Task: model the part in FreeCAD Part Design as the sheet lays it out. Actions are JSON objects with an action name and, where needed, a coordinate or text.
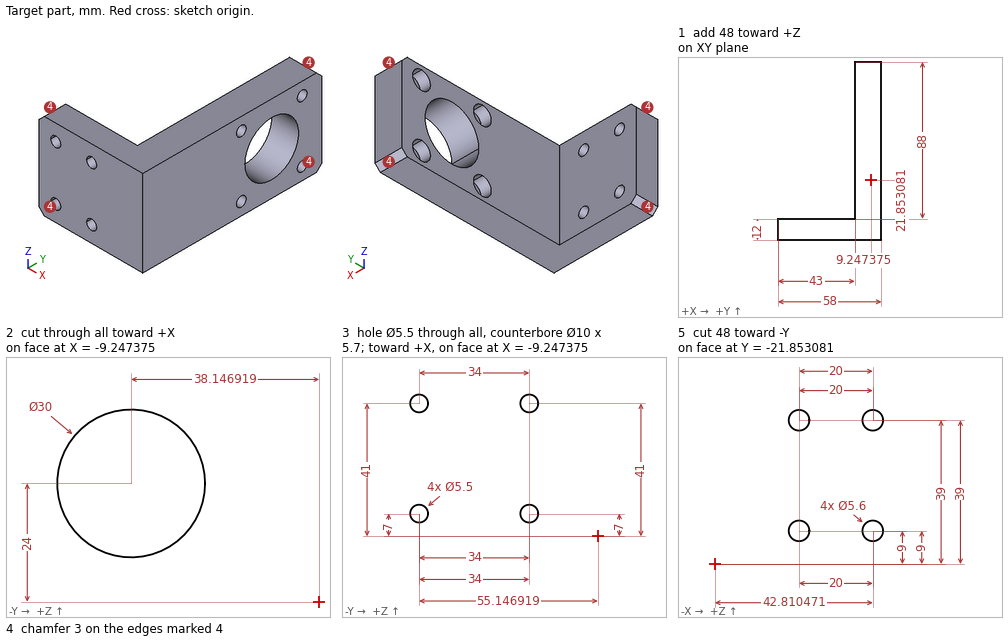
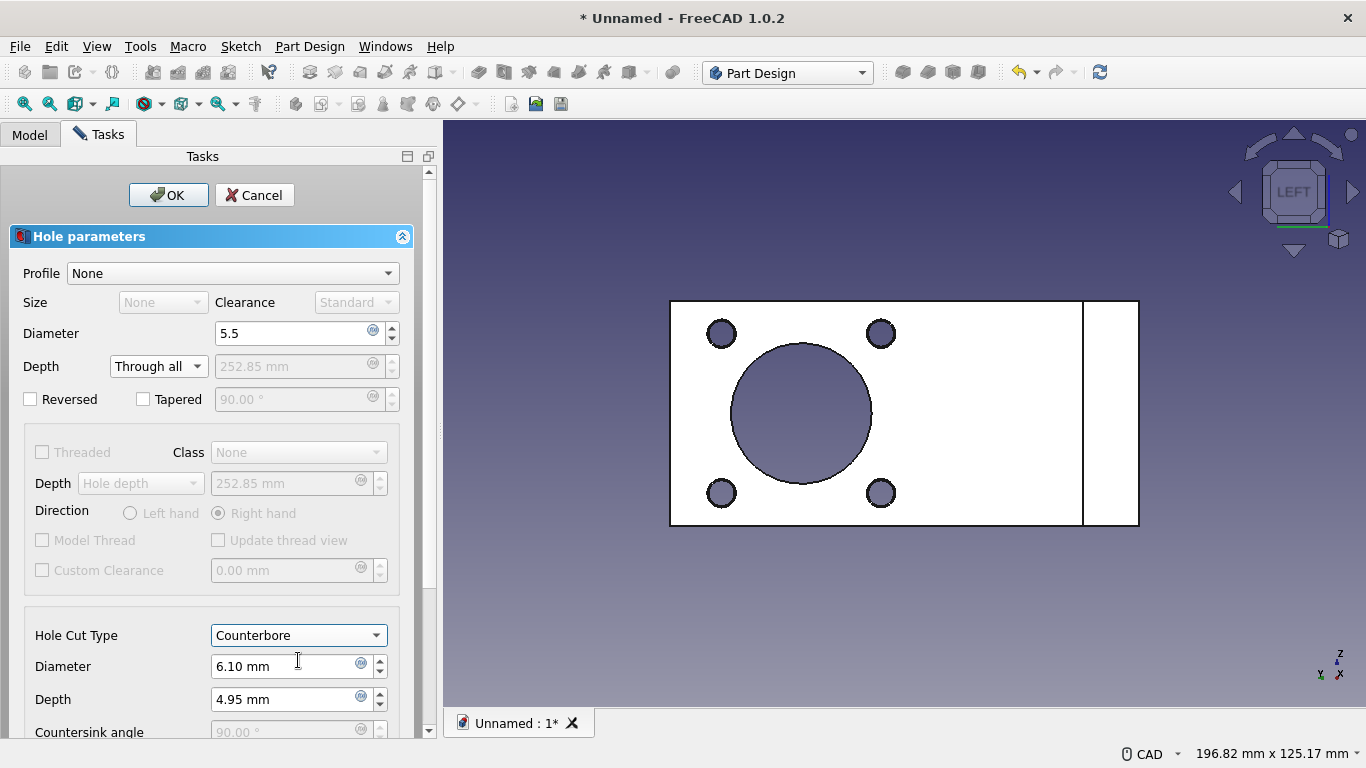
{"action": "triple_click", "coordinate": [292, 666]}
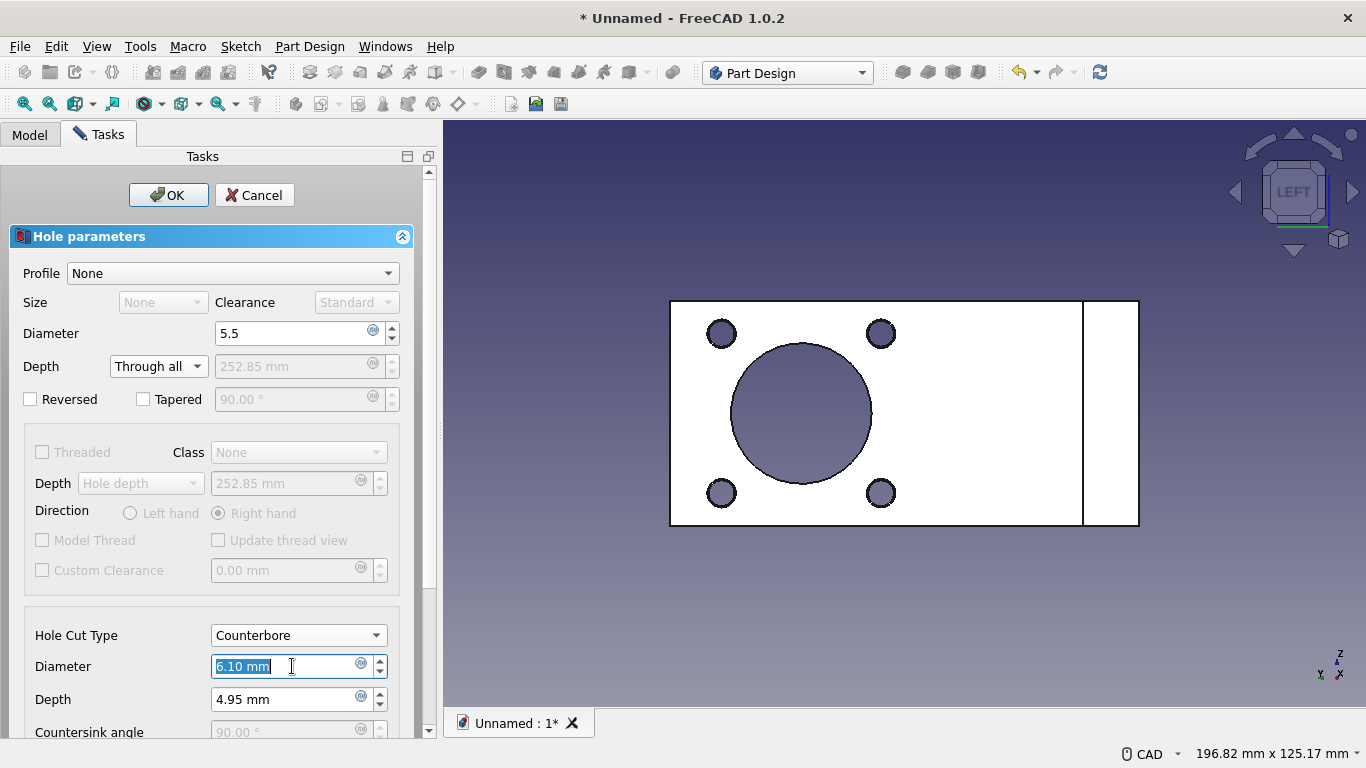
{"action": "type", "text": "10"}
{"action": "key", "text": "Tab"}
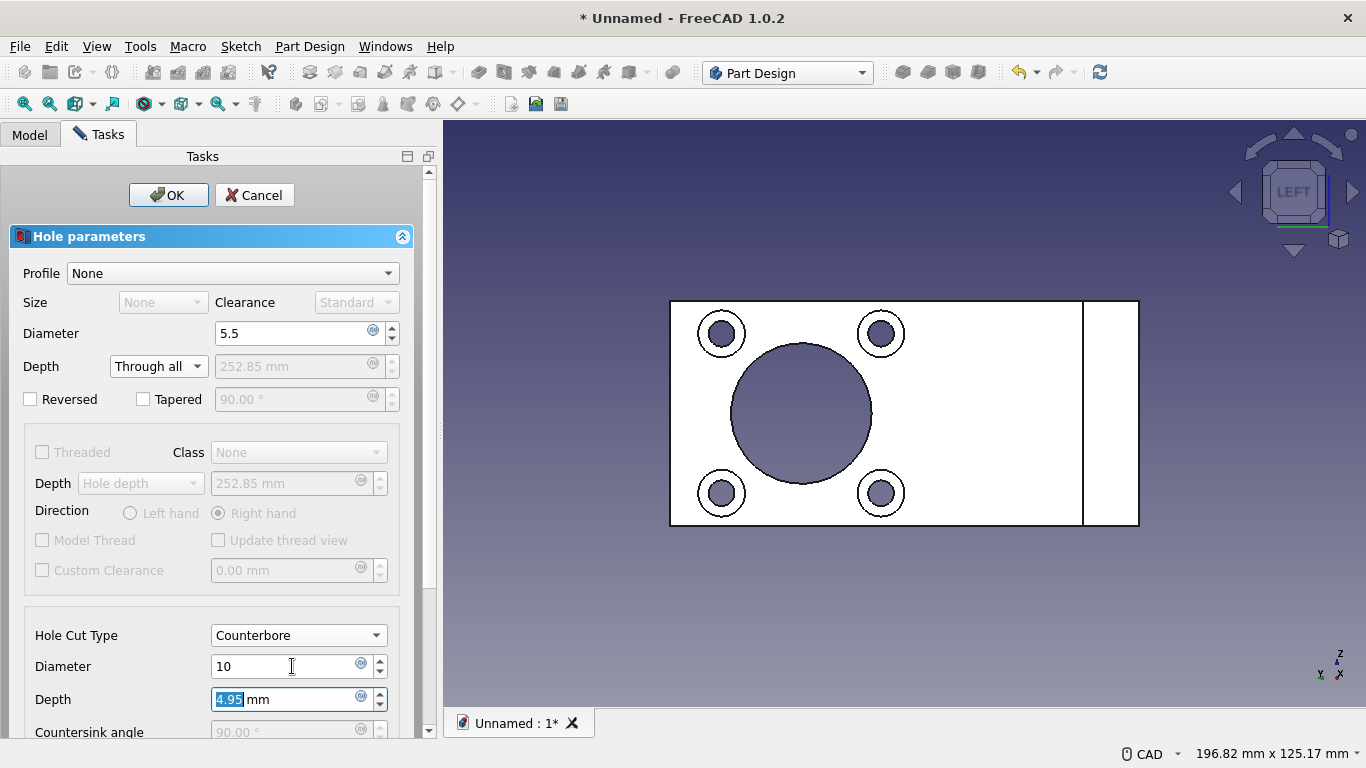
{"action": "type", "text": "5.7"}
{"action": "key", "text": "Tab"}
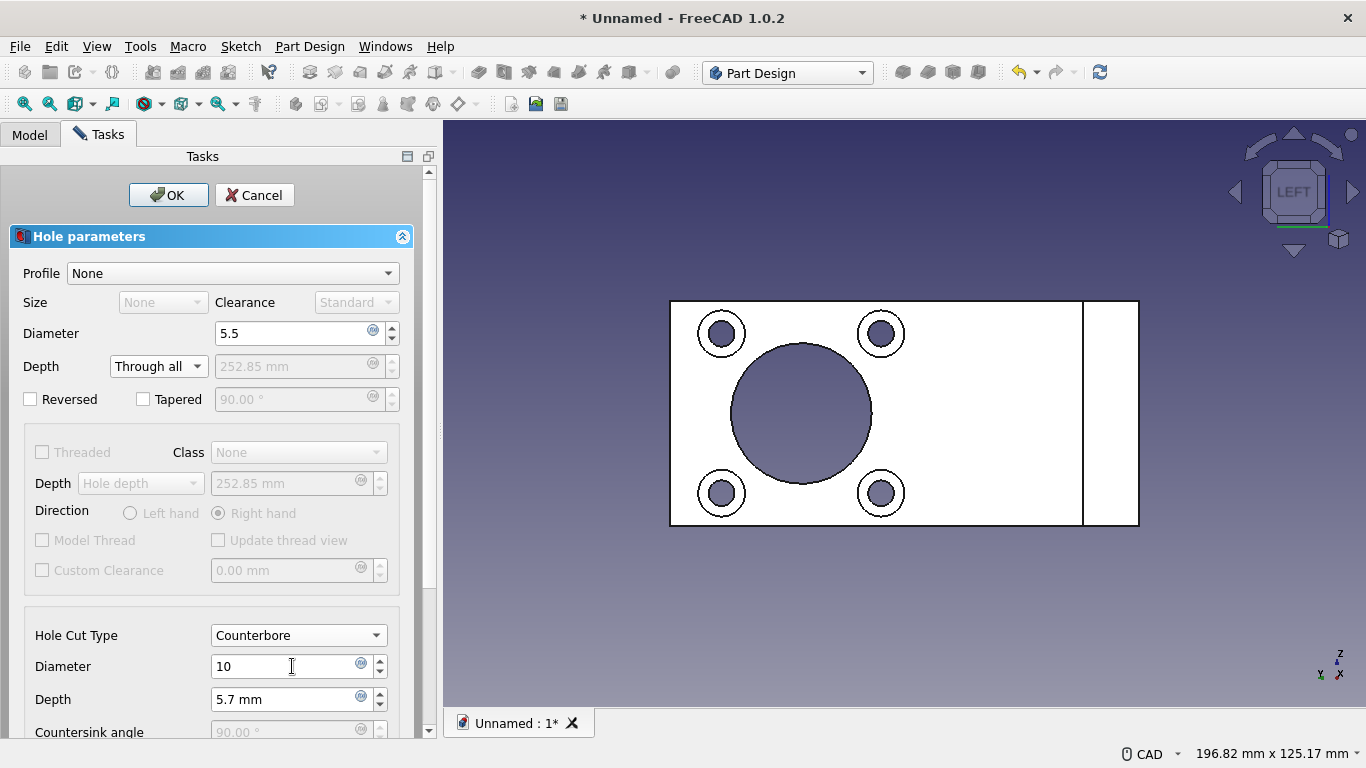
{"action": "left_click", "coordinate": [169, 195]}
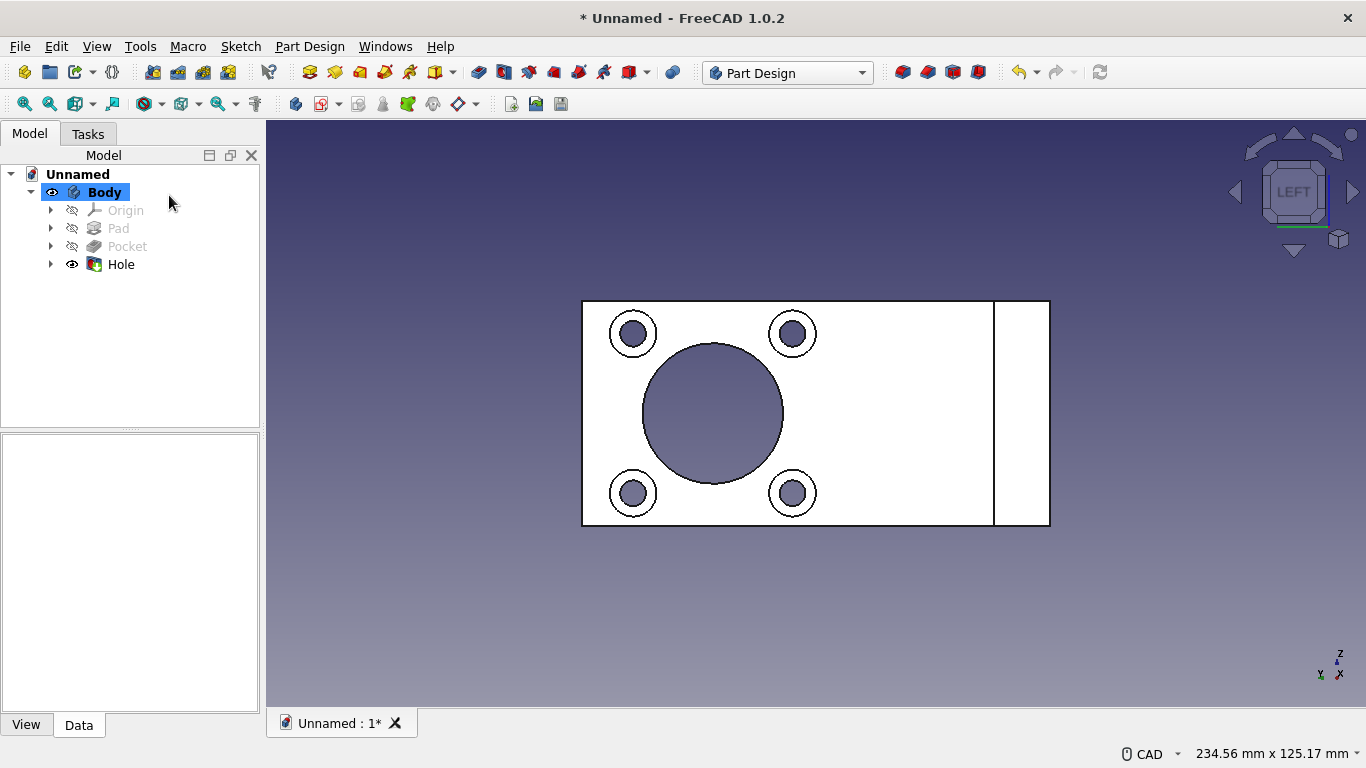
{"action": "left_click", "coordinate": [25, 104]}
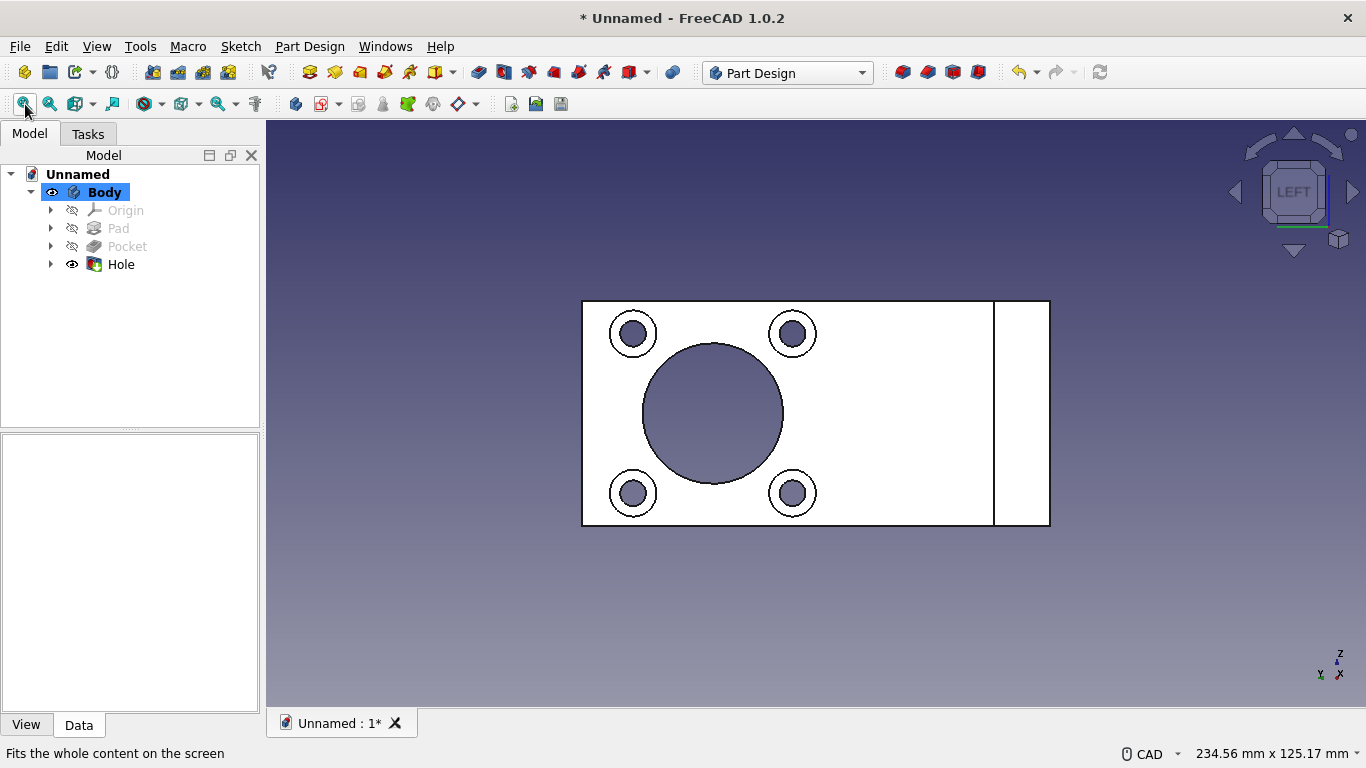
{"action": "left_click", "coordinate": [1022, 300]}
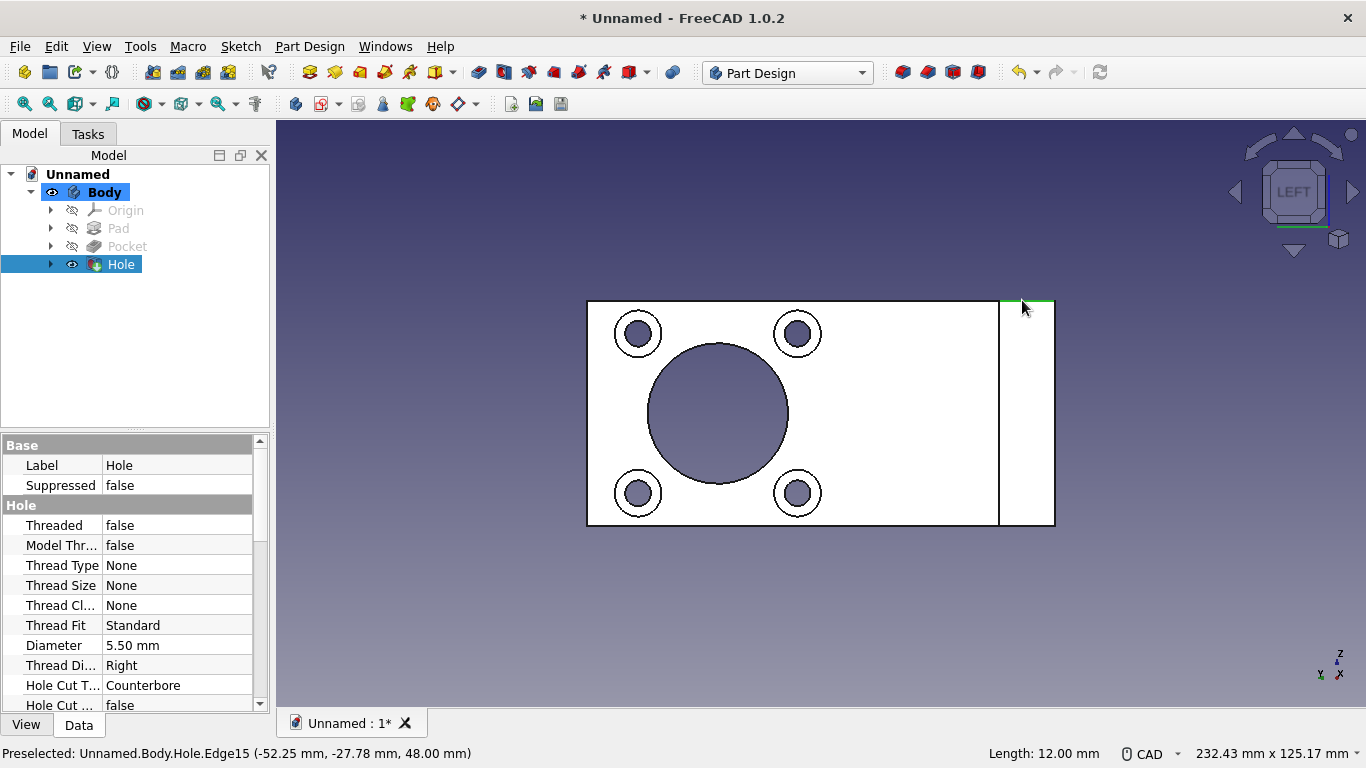
{"action": "left_click", "coordinate": [1027, 525], "text": "ctrl"}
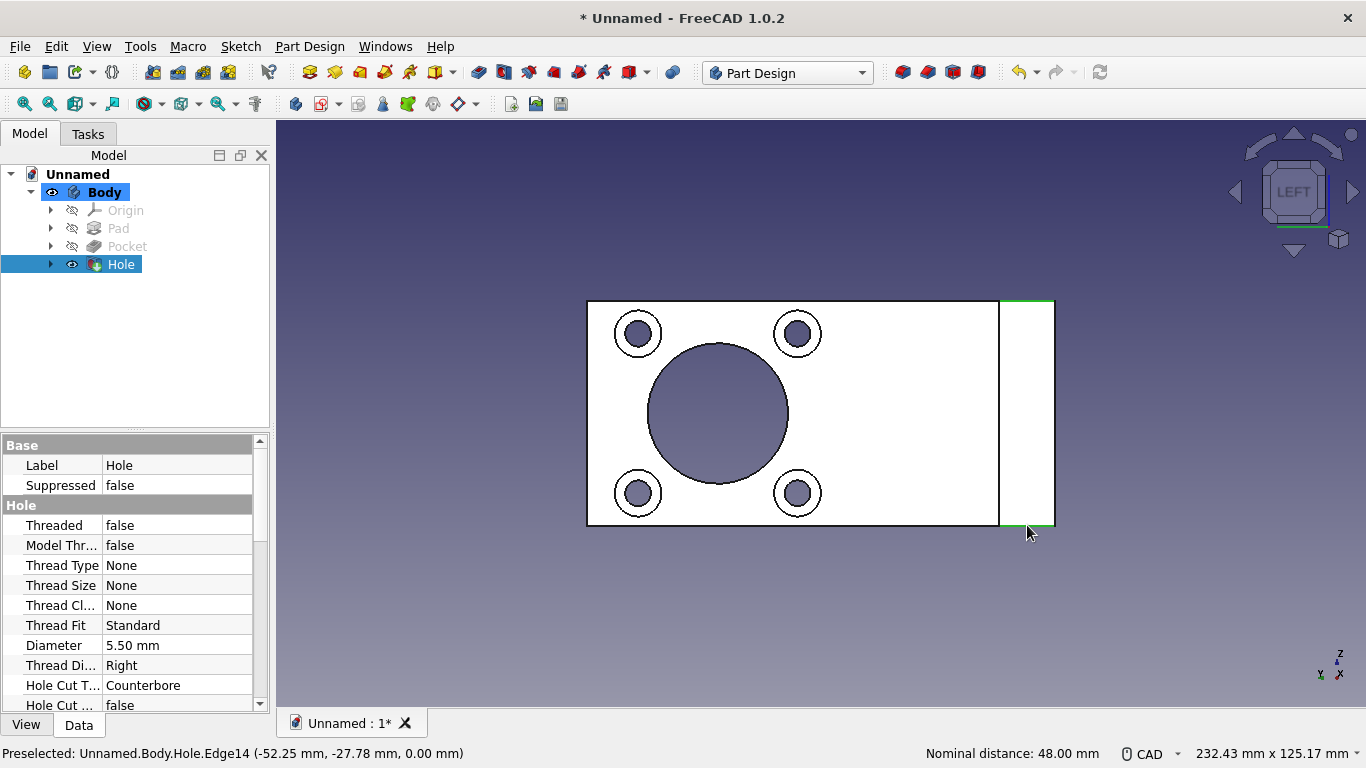
{"action": "key", "text": "0"}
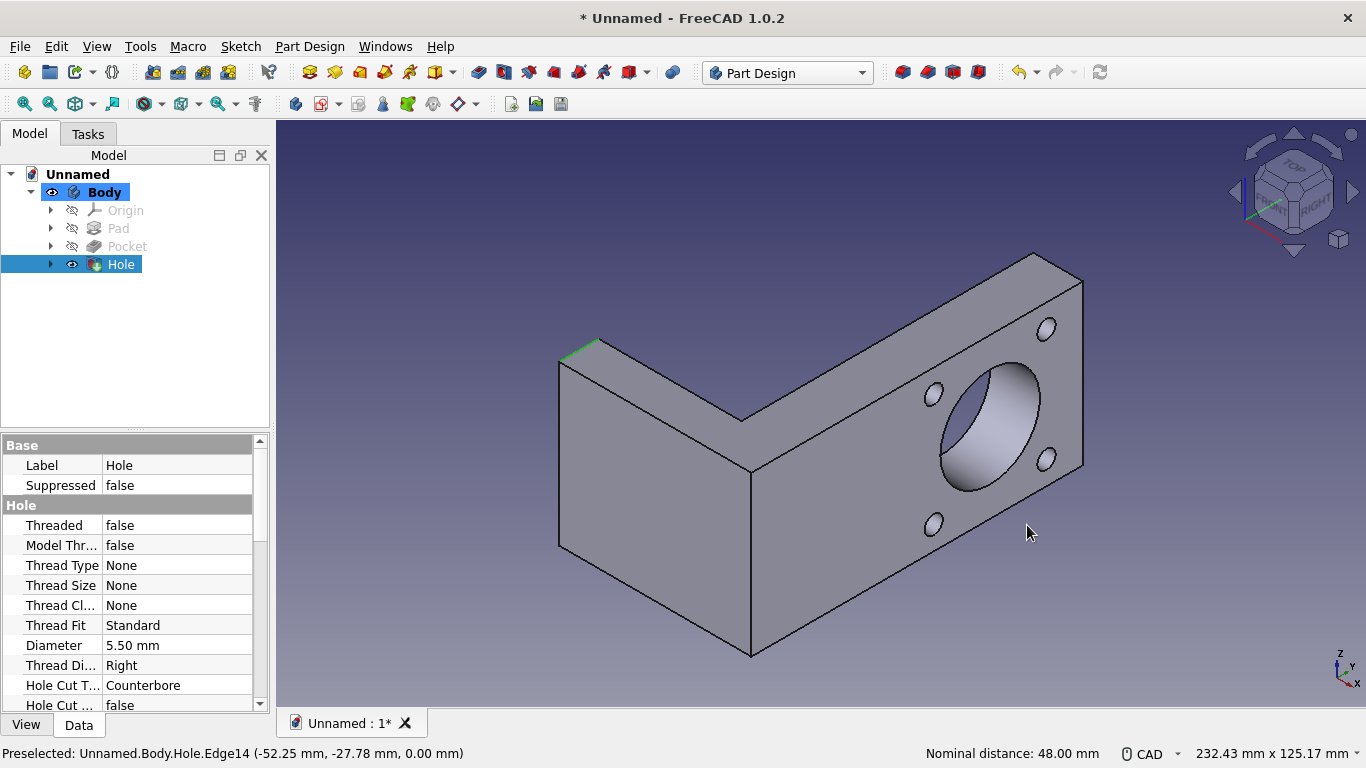
{"action": "key", "text": "2"}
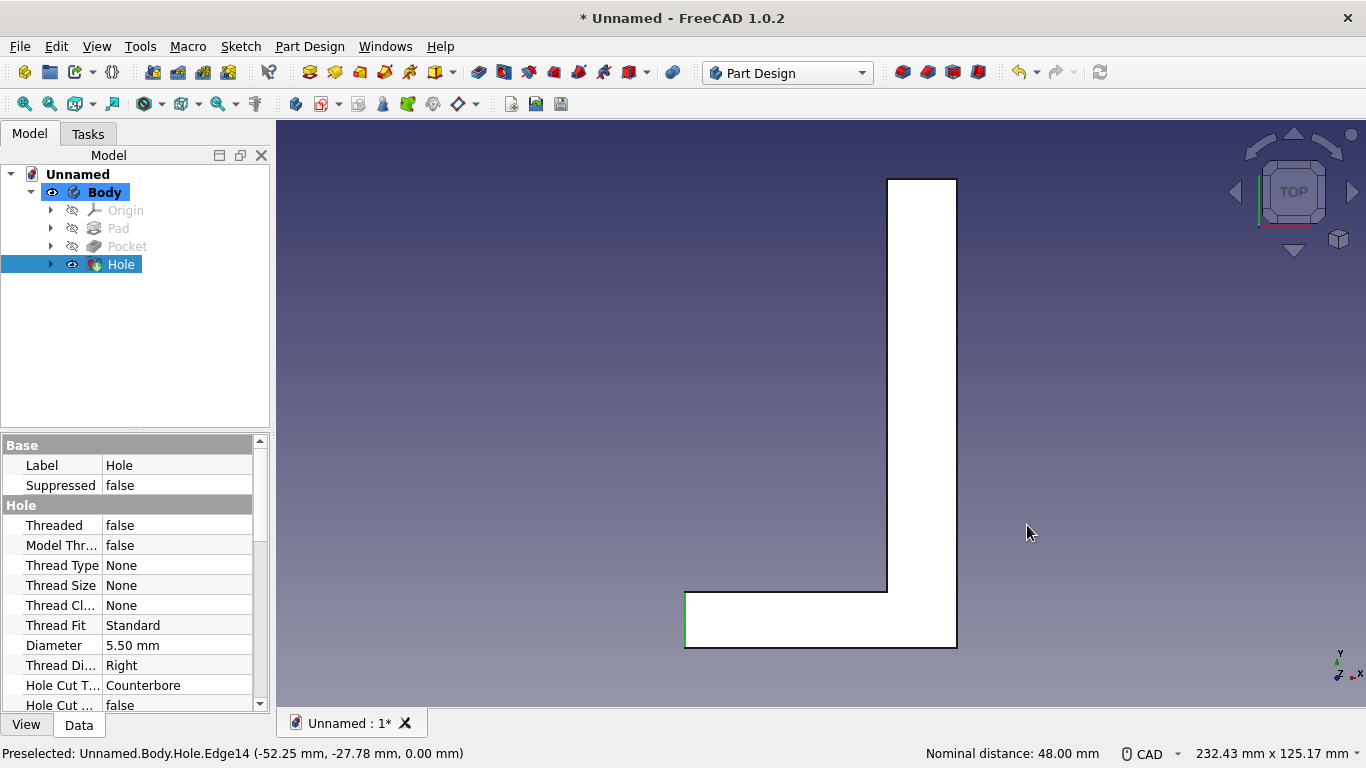
{"action": "left_click", "coordinate": [922, 178], "text": "ctrl"}